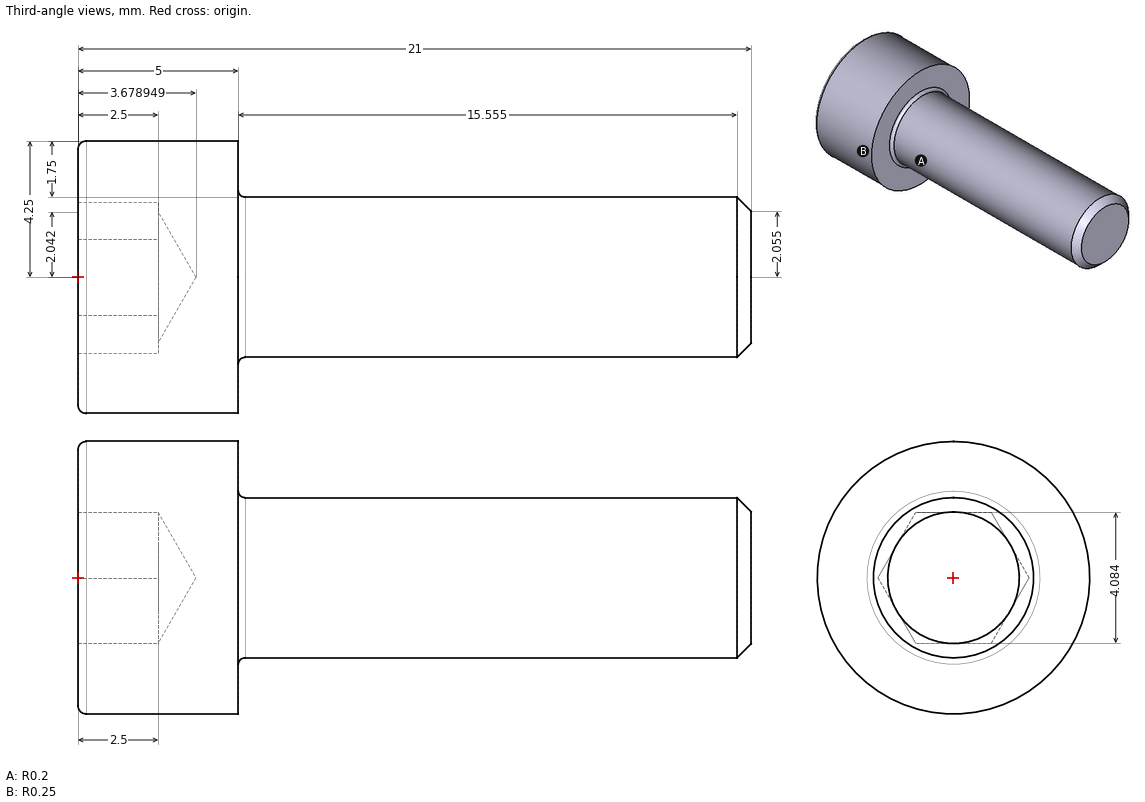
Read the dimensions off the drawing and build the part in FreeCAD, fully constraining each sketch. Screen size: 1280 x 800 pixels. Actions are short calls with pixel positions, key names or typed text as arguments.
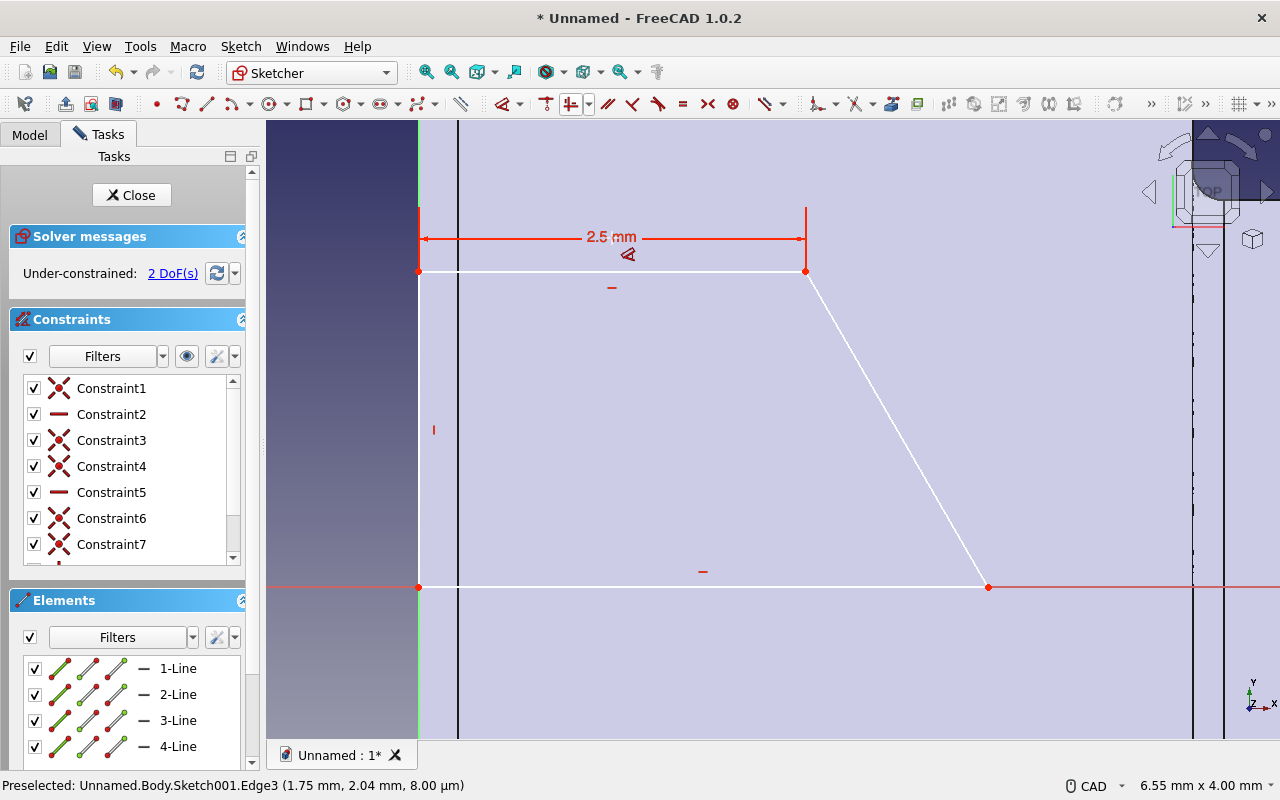
click(419, 367)
click(385, 430)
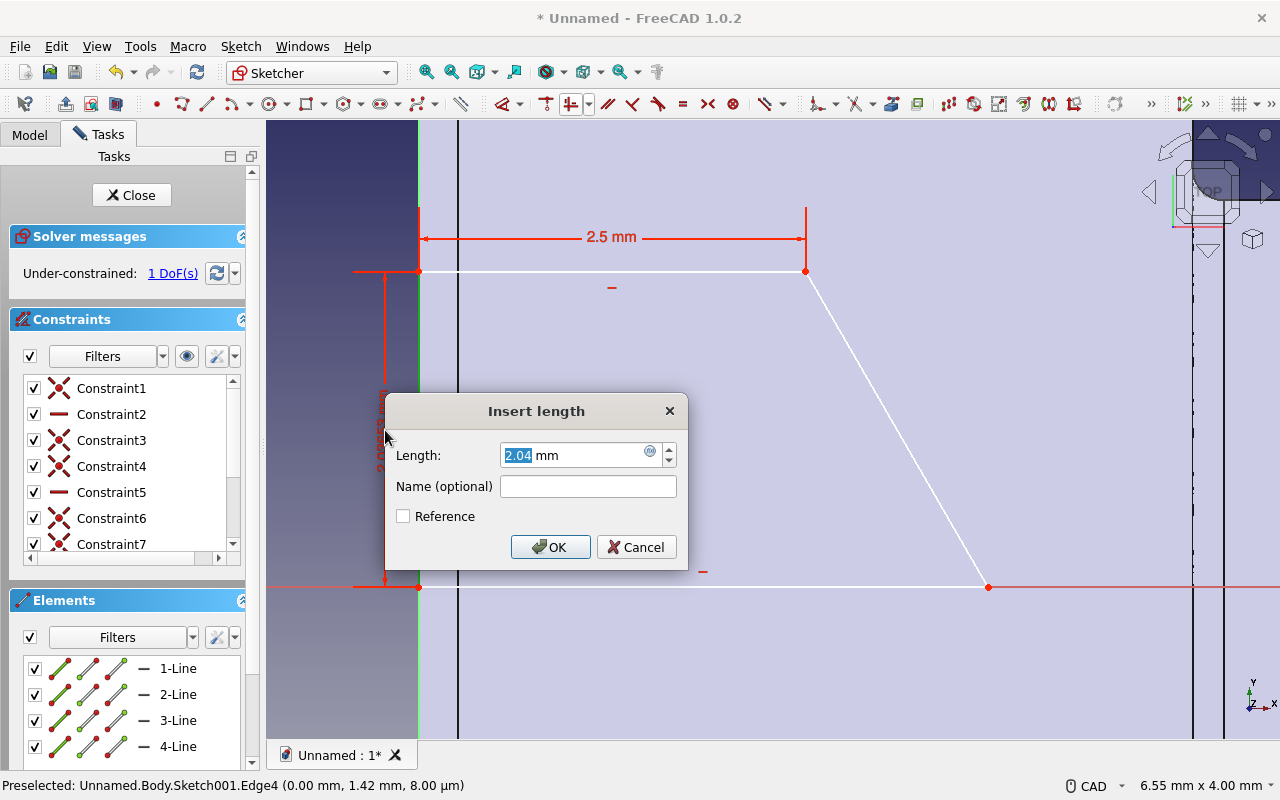
text(2.042)
key(Return)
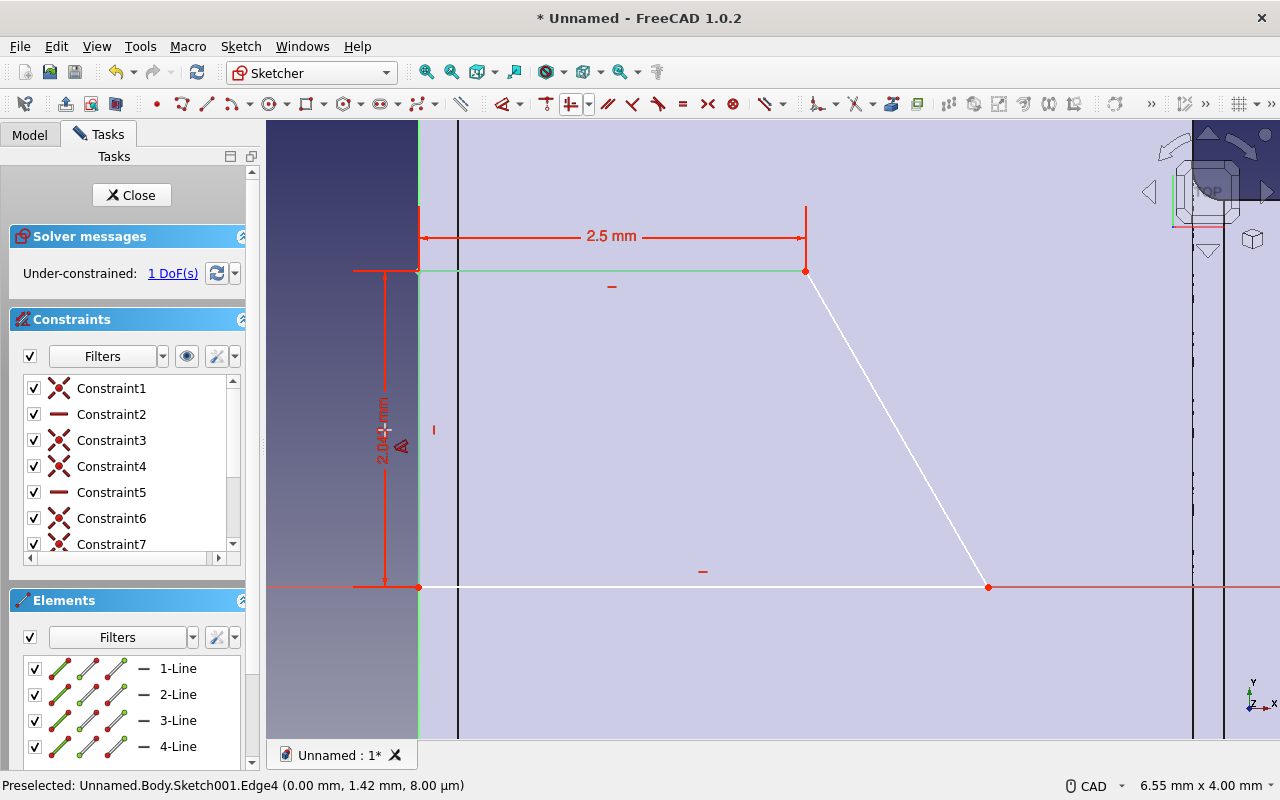
click(590, 587)
click(703, 621)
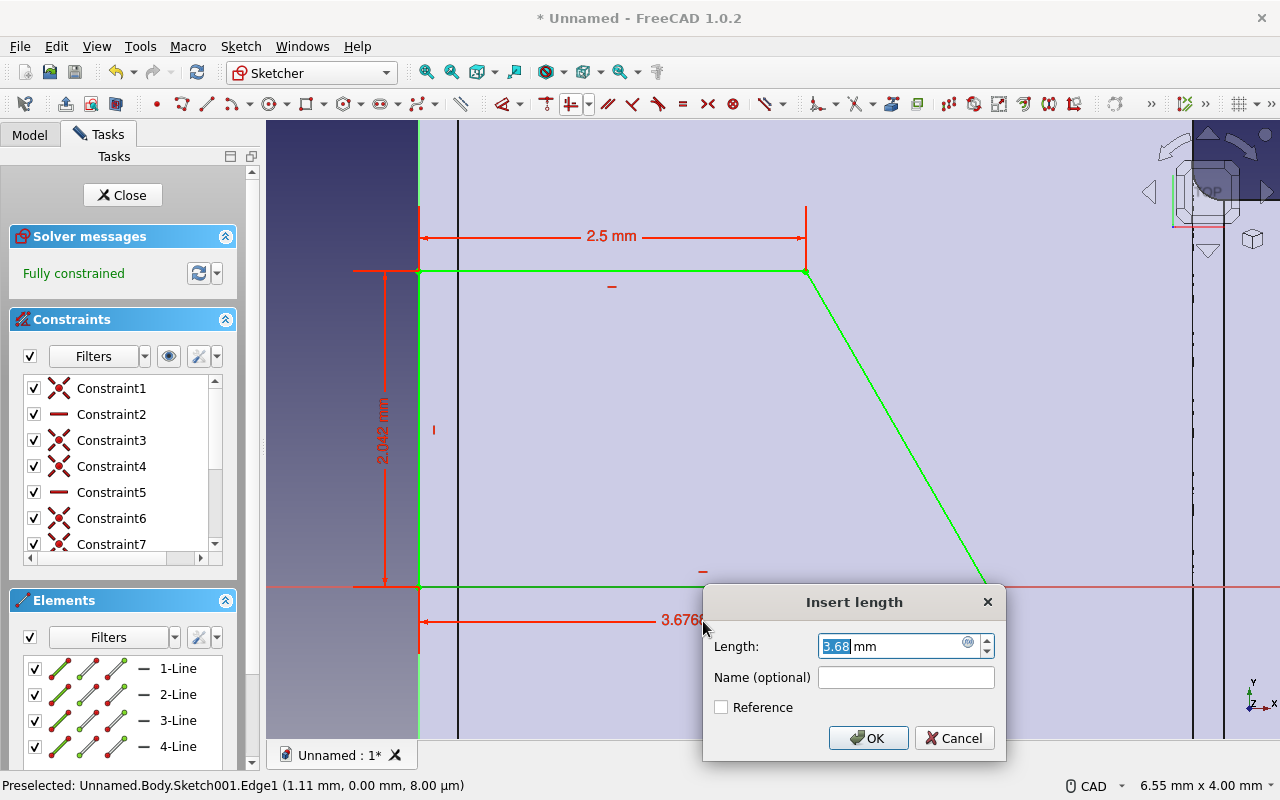
text(3.678949)
key(Return)
key(Escape)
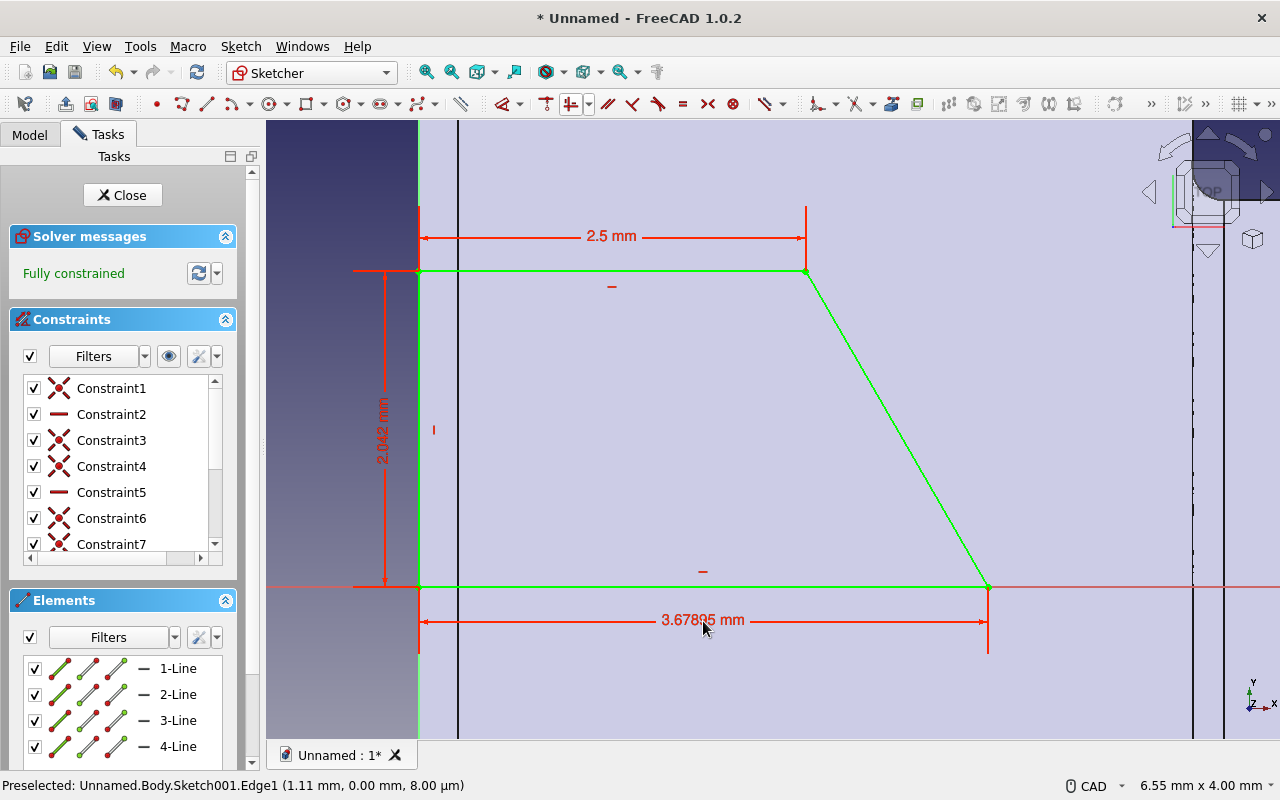
click(123, 195)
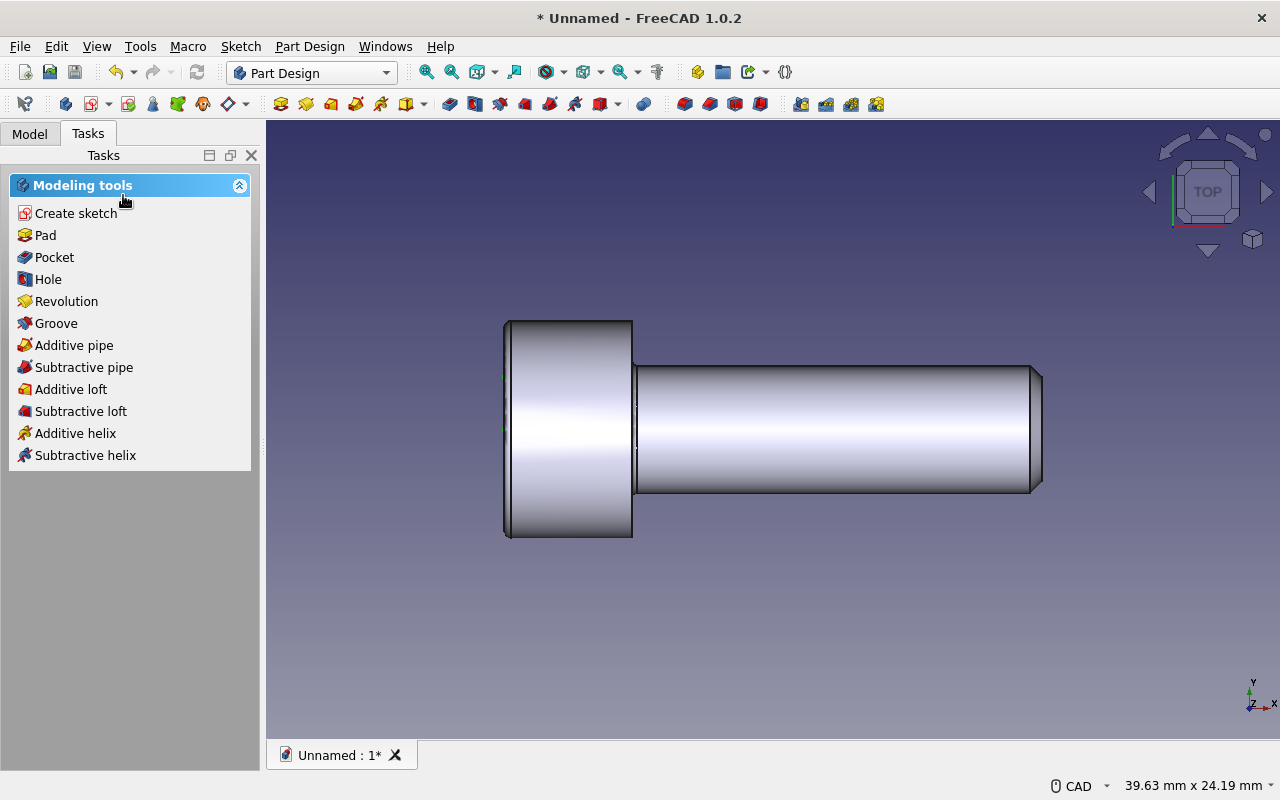
click(500, 104)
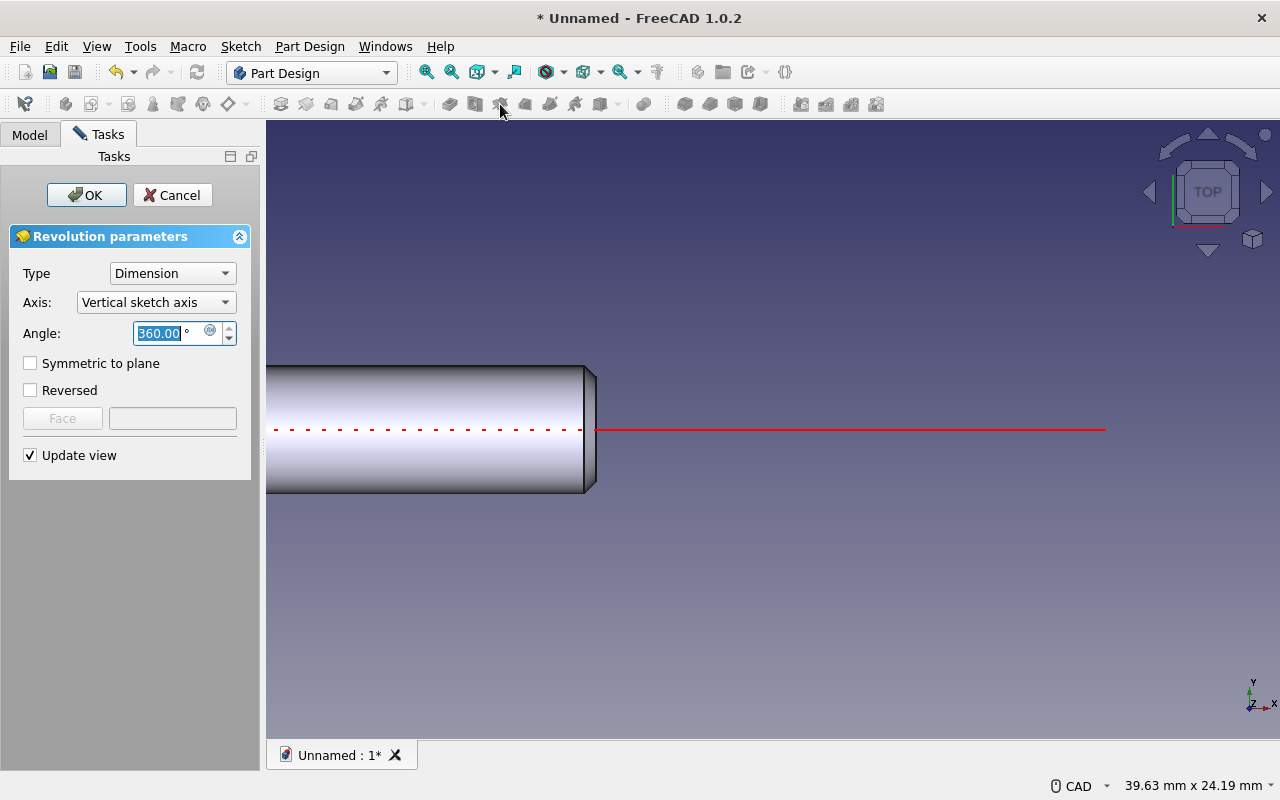
click(157, 302)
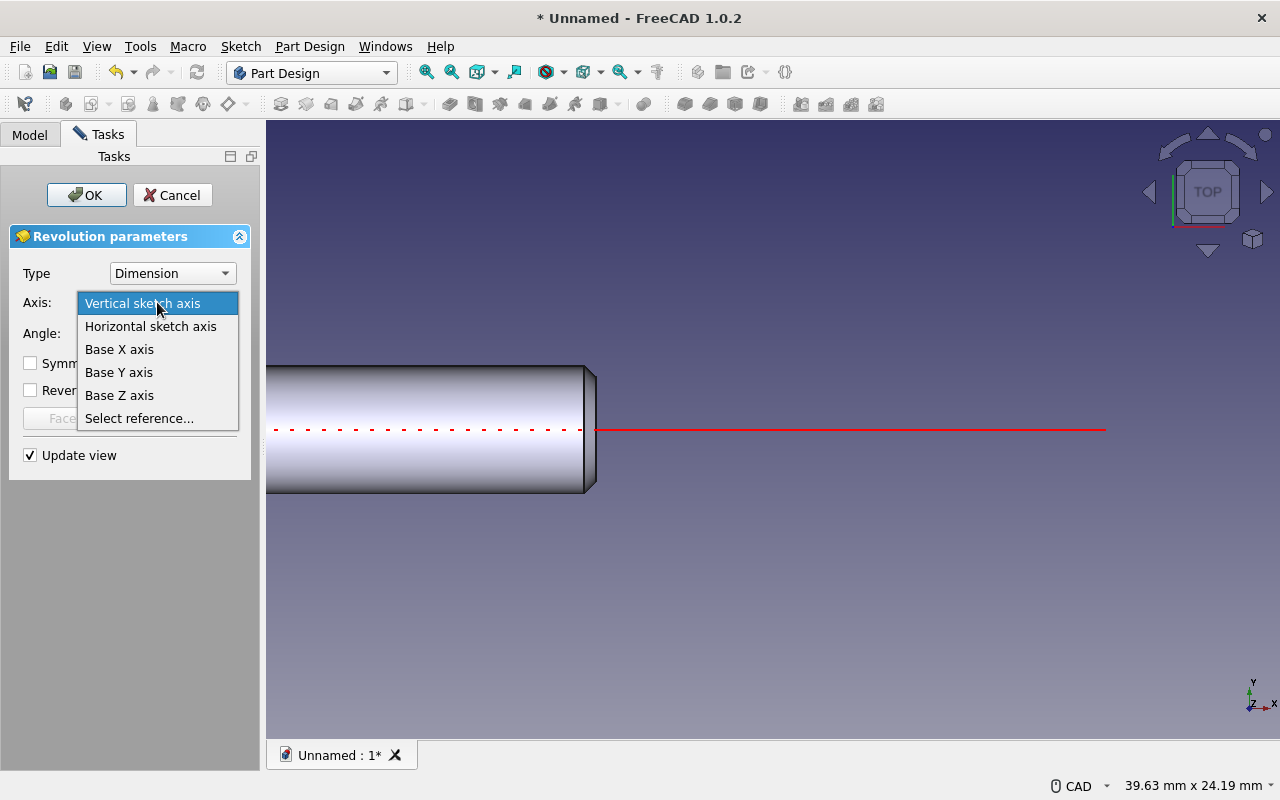
click(156, 326)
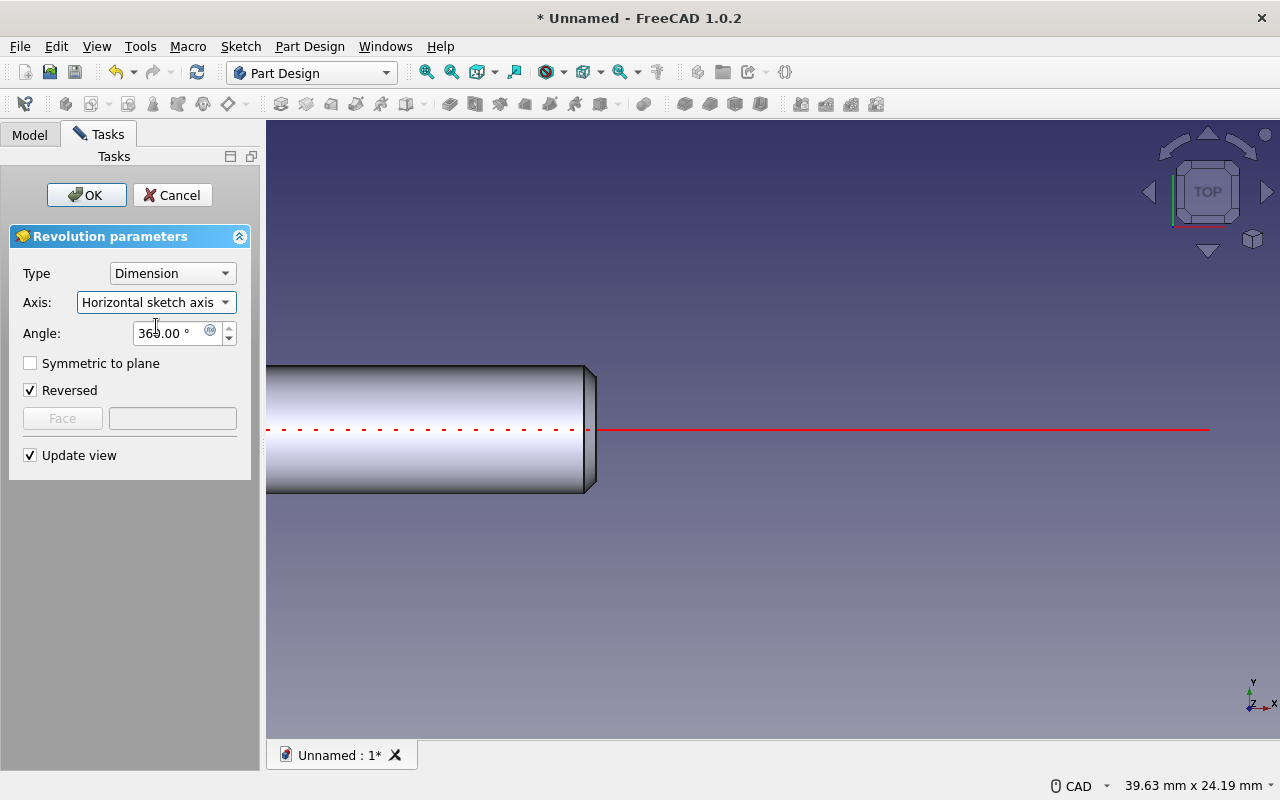
click(87, 195)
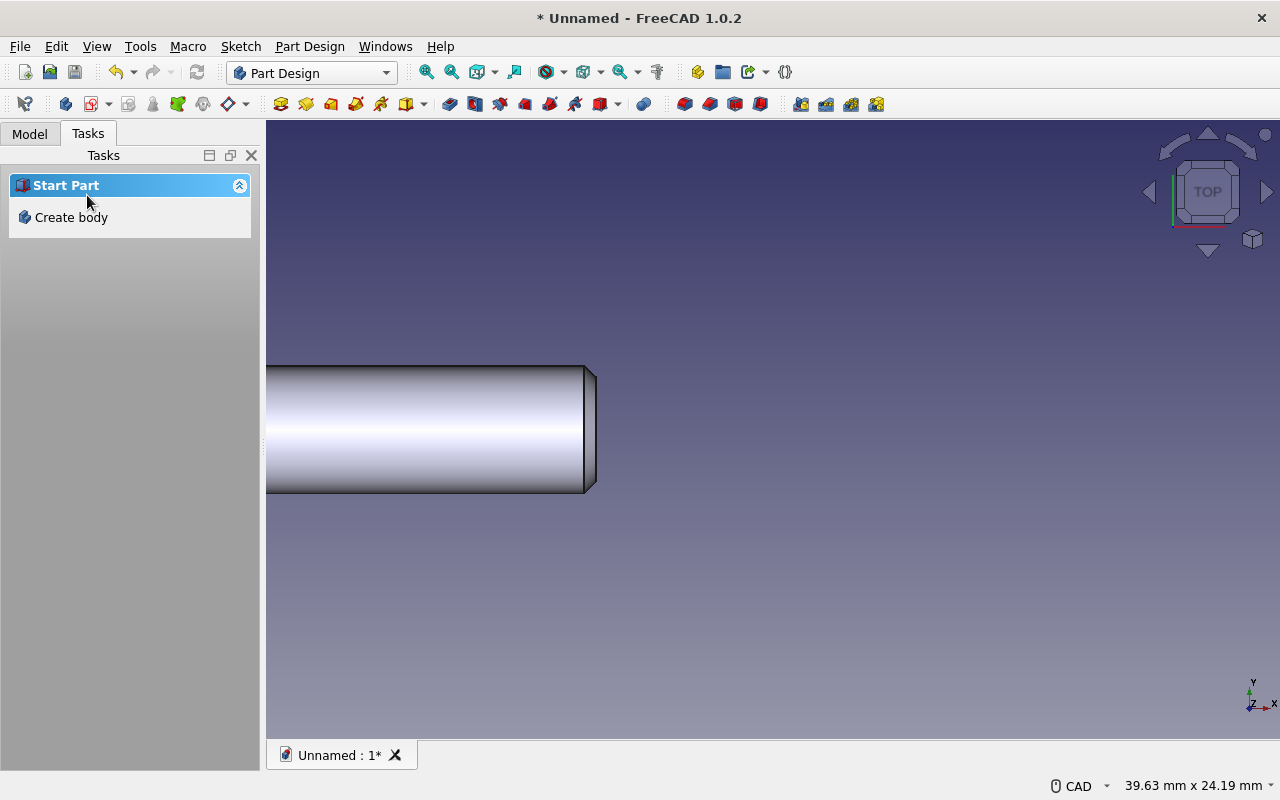
click(427, 72)